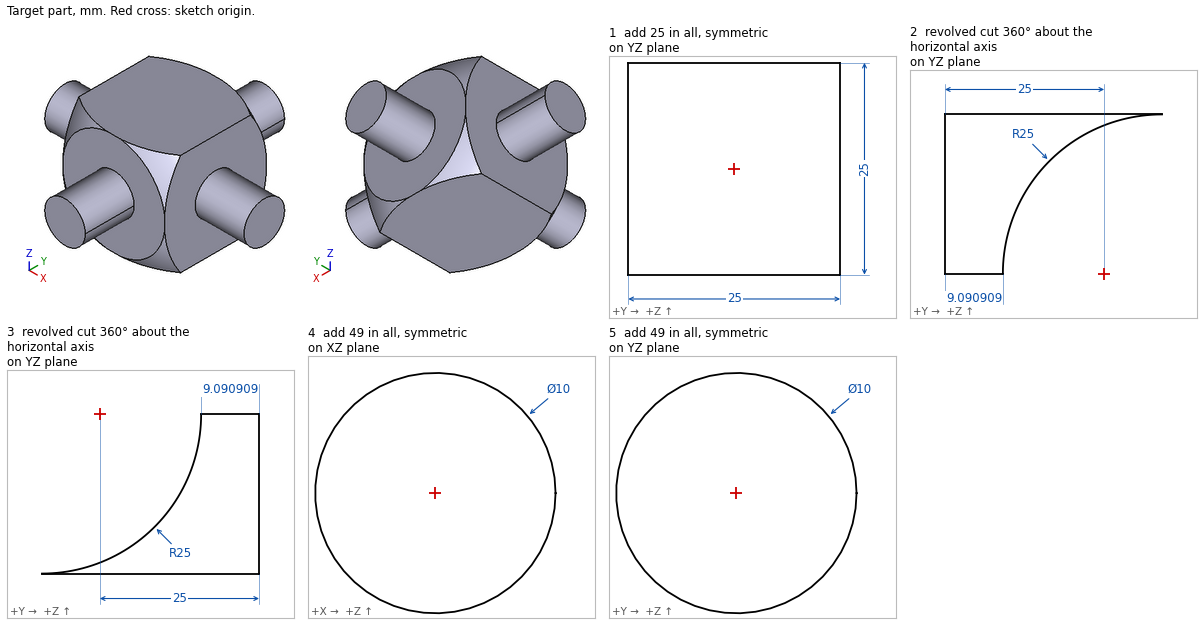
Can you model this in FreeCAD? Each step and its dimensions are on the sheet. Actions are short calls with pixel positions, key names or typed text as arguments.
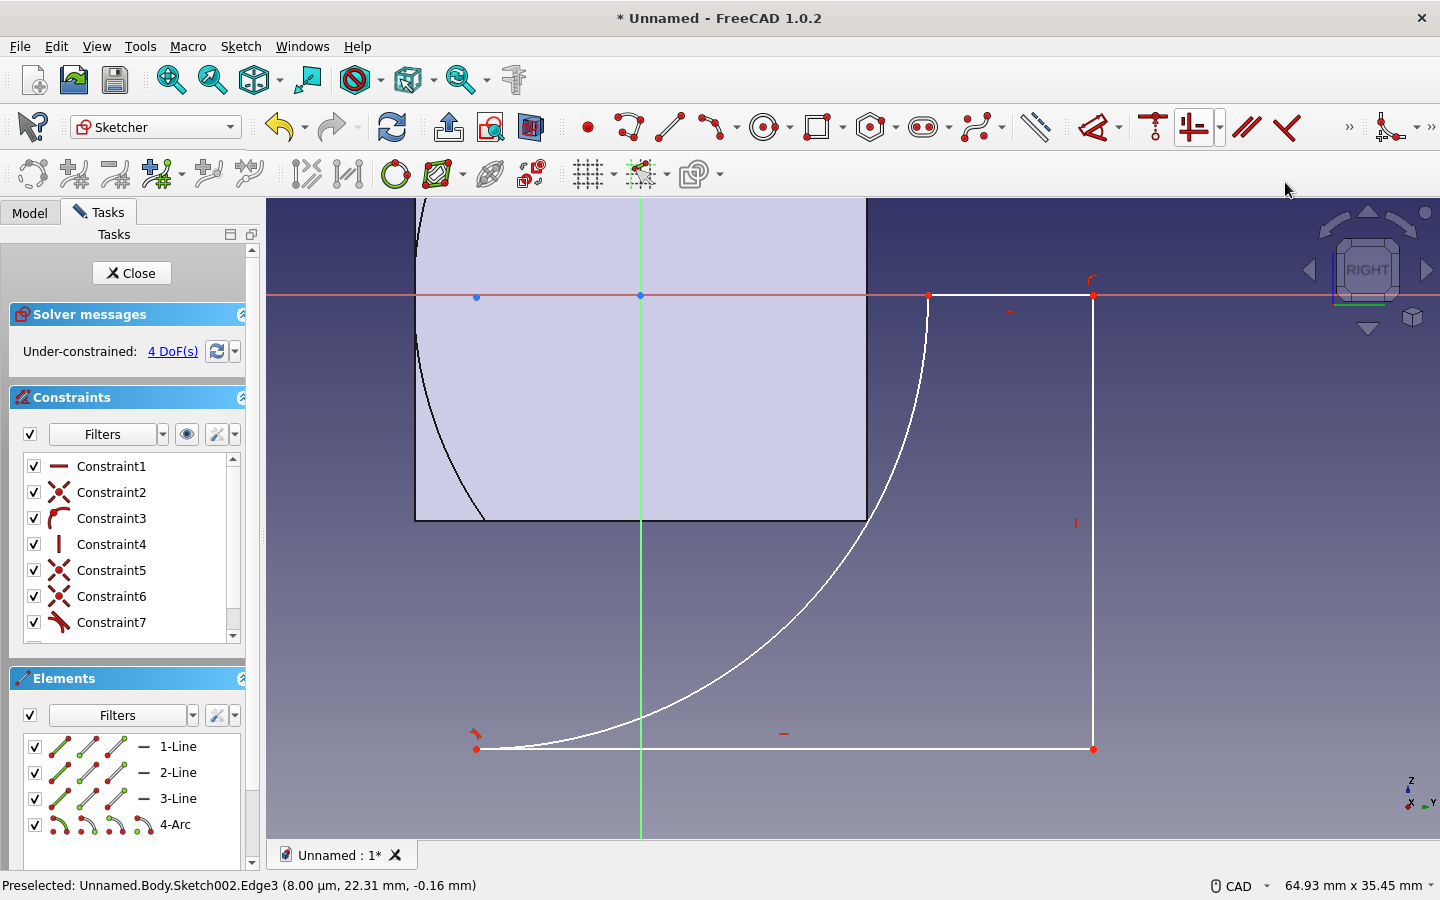
click(476, 297)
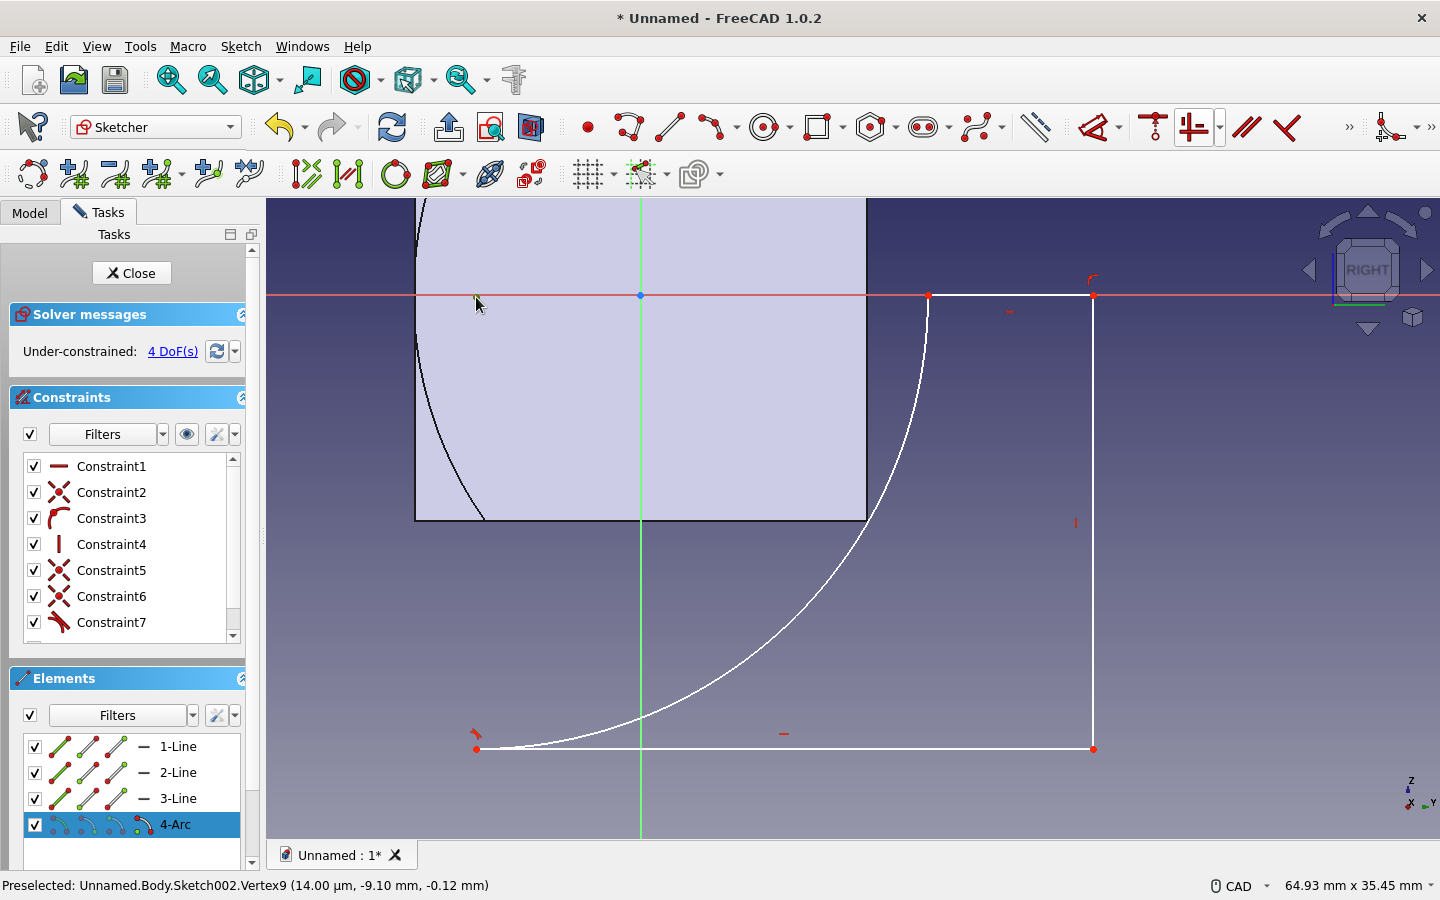
click(364, 295)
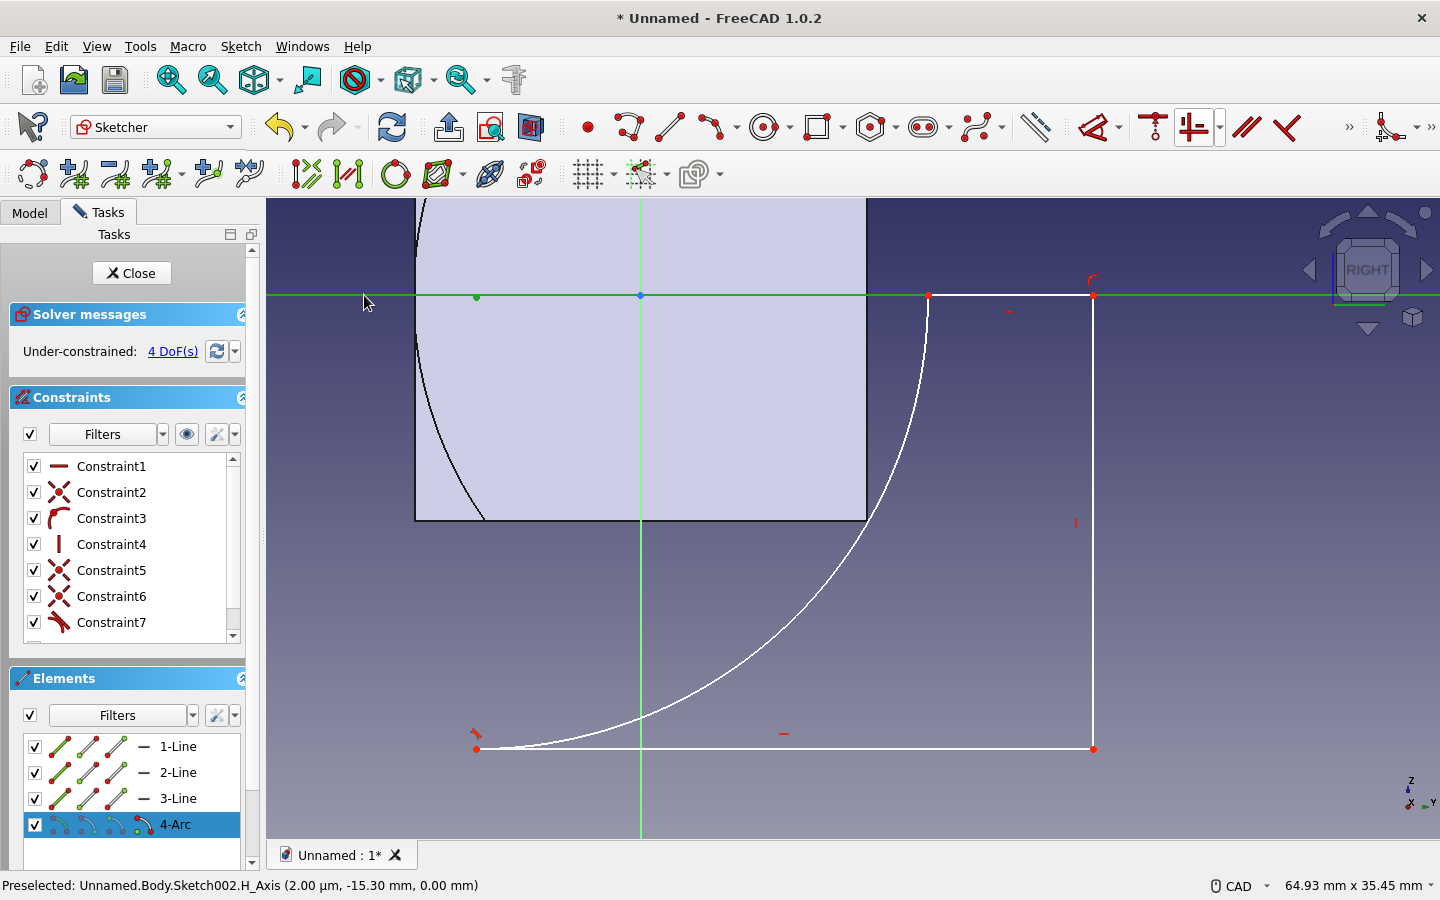
click(1153, 128)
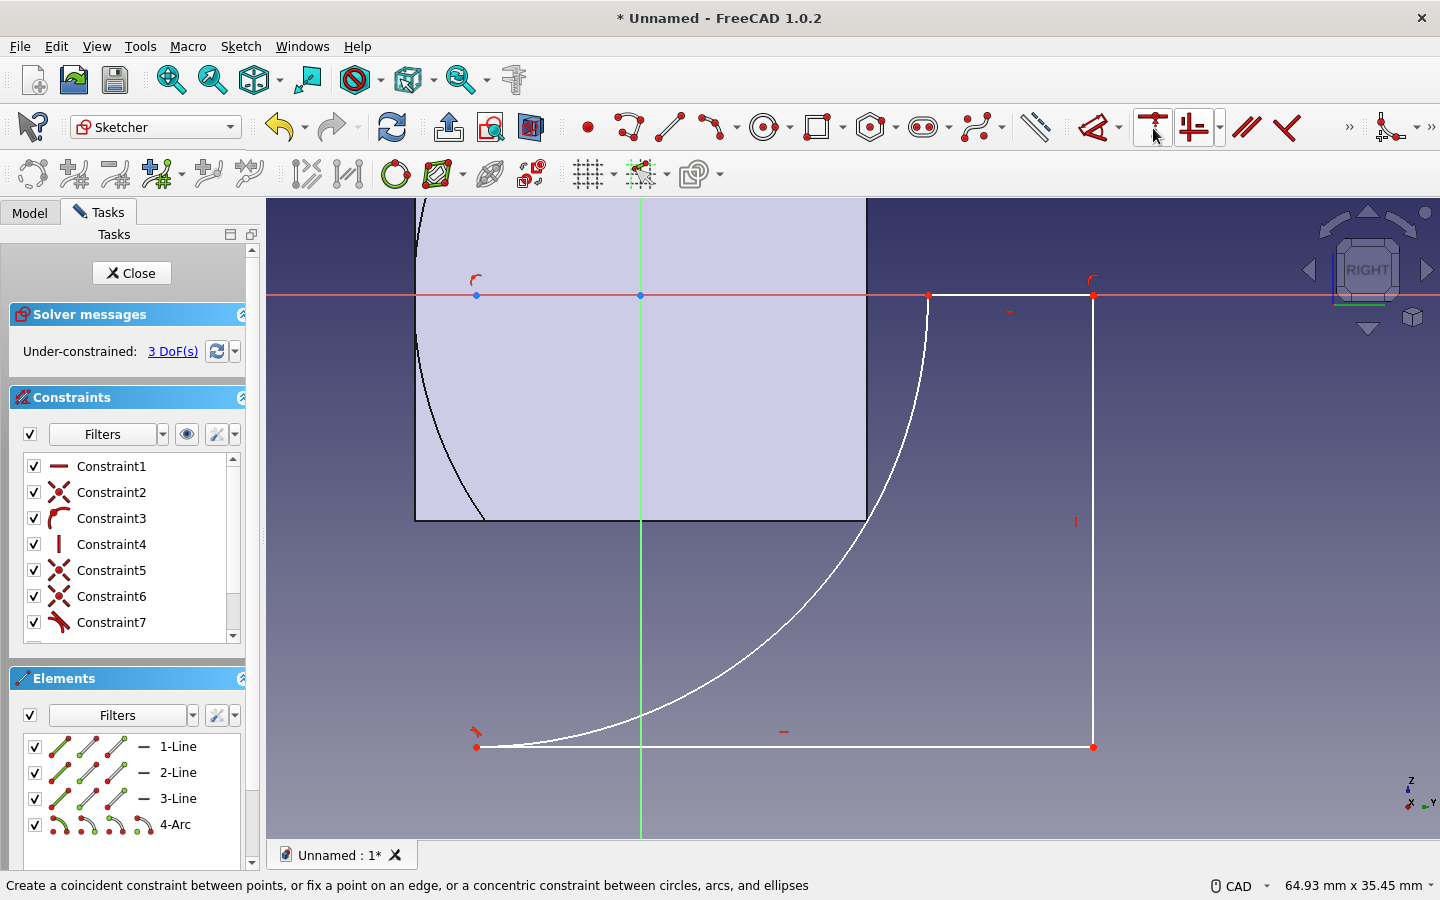
key(d)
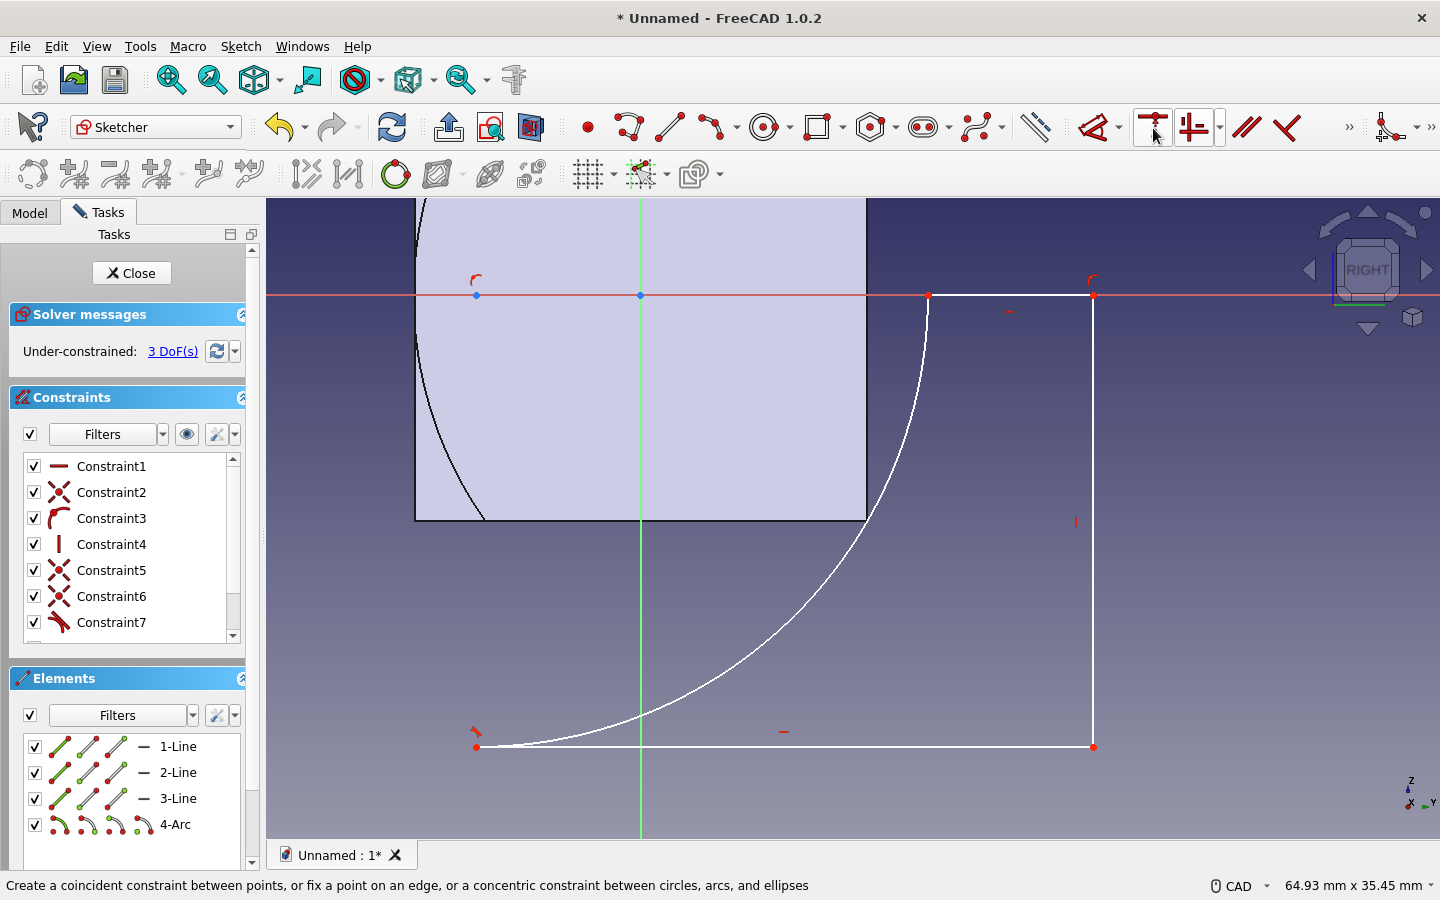
click(681, 698)
click(696, 727)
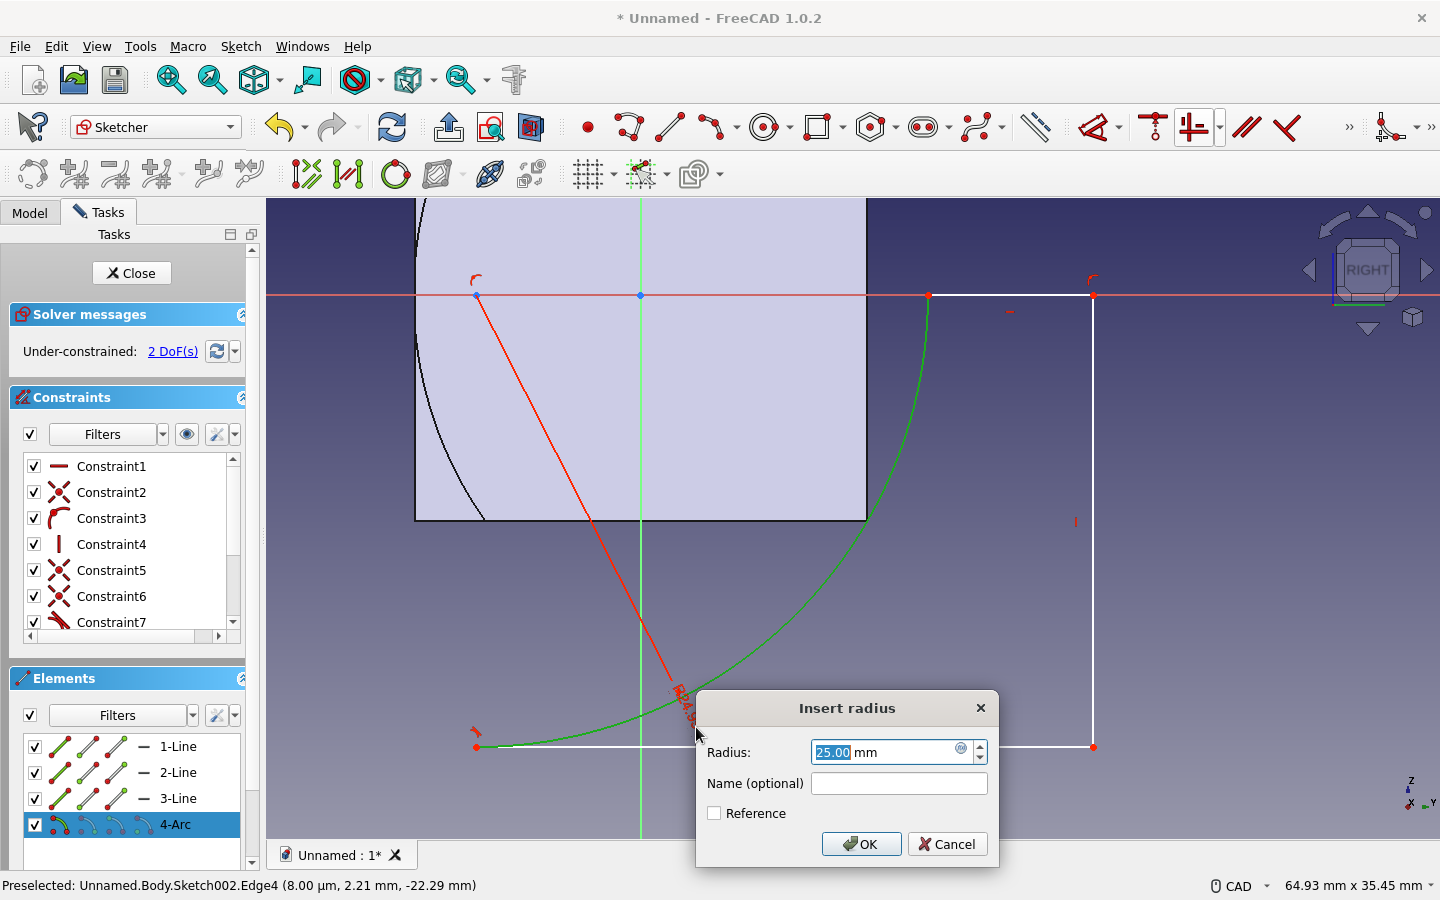
text(25)
key(Return)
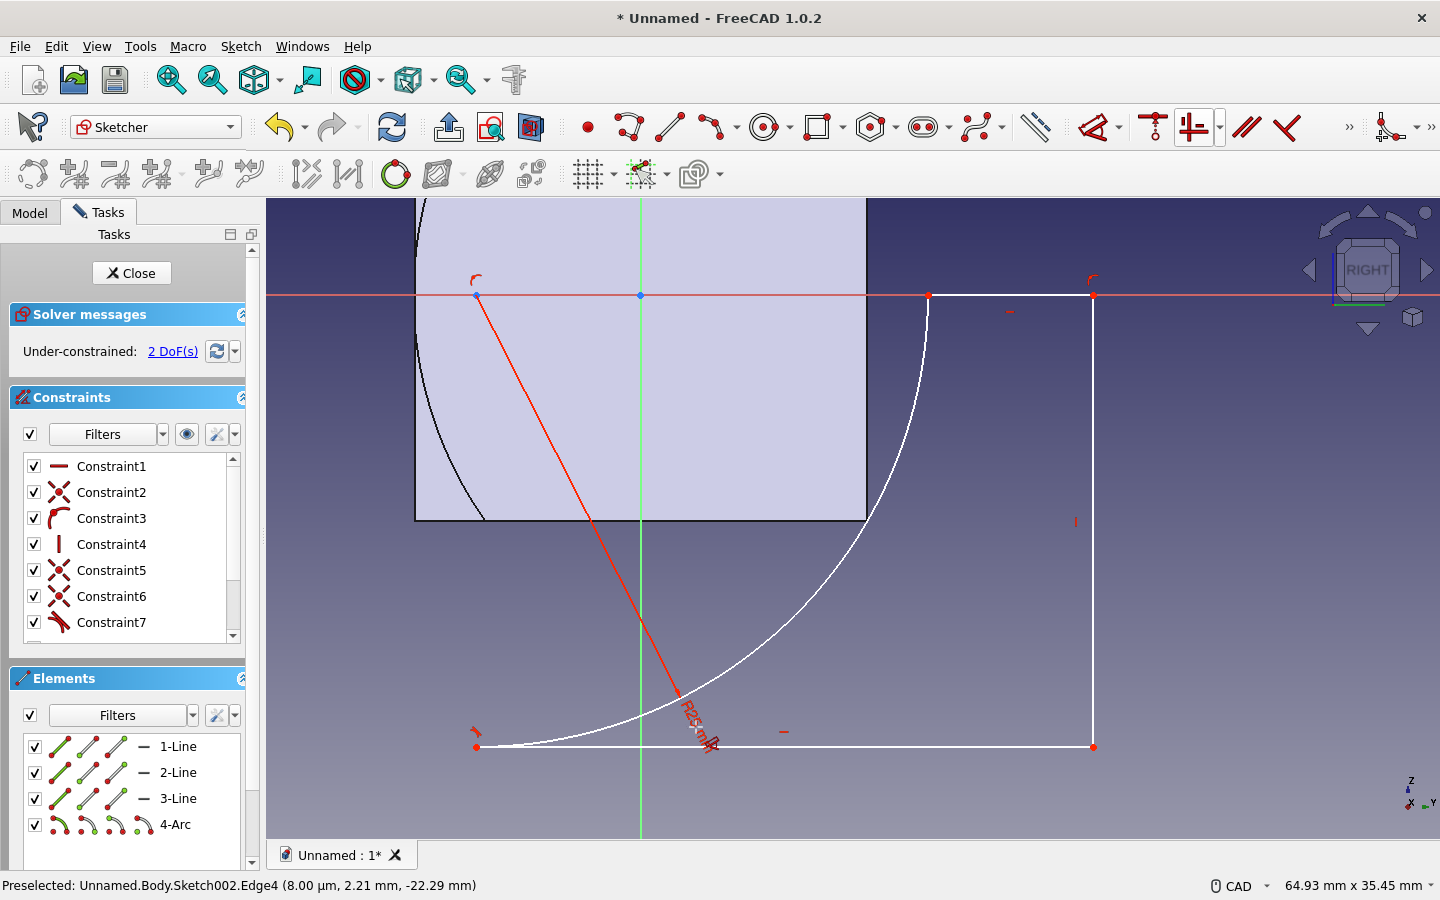
click(1093, 747)
click(867, 781)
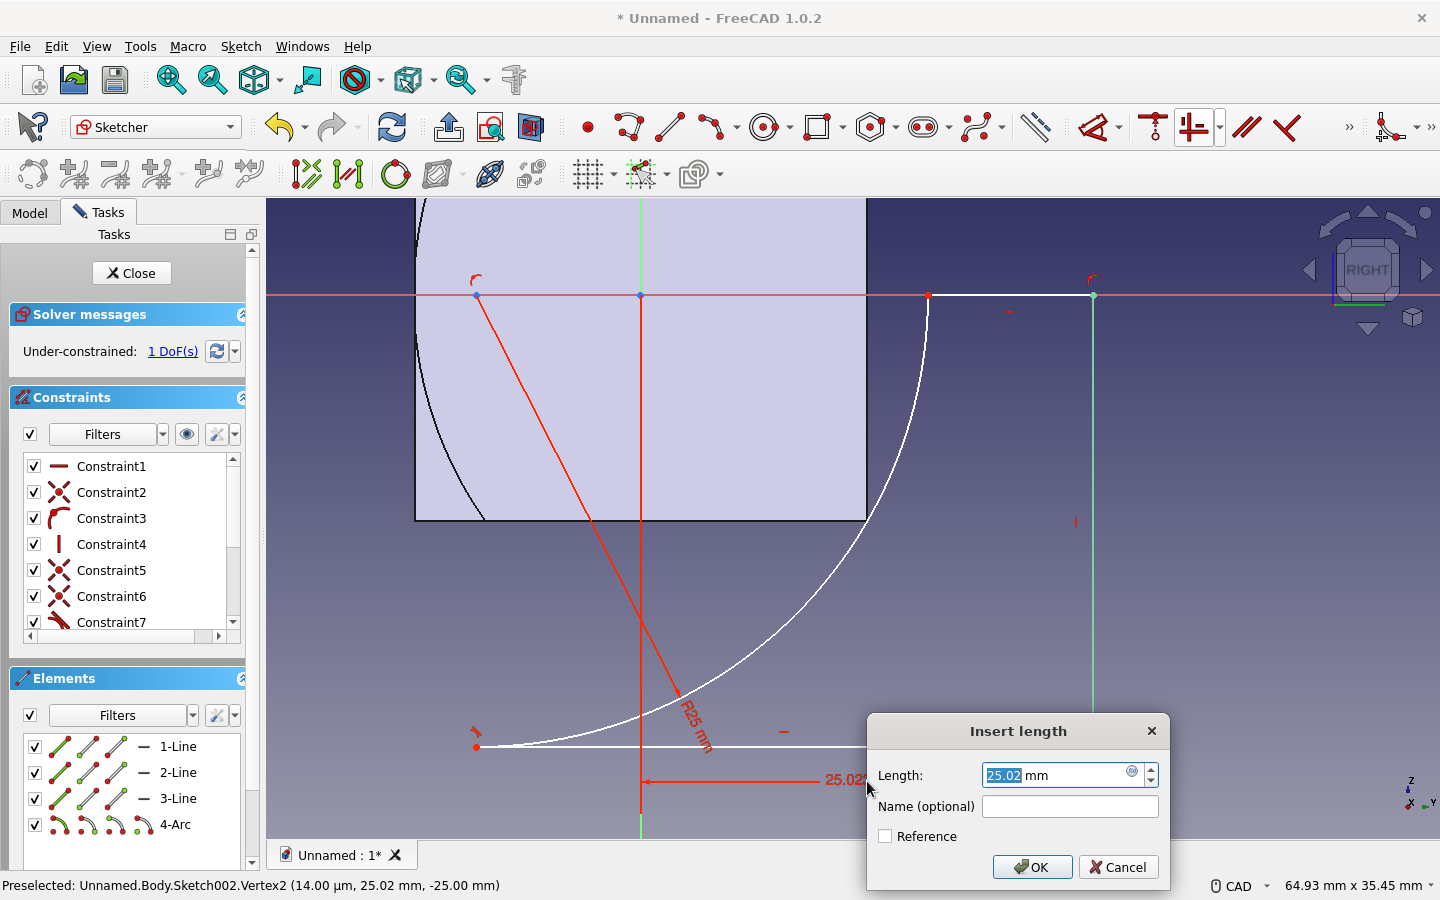
text(25)
key(Return)